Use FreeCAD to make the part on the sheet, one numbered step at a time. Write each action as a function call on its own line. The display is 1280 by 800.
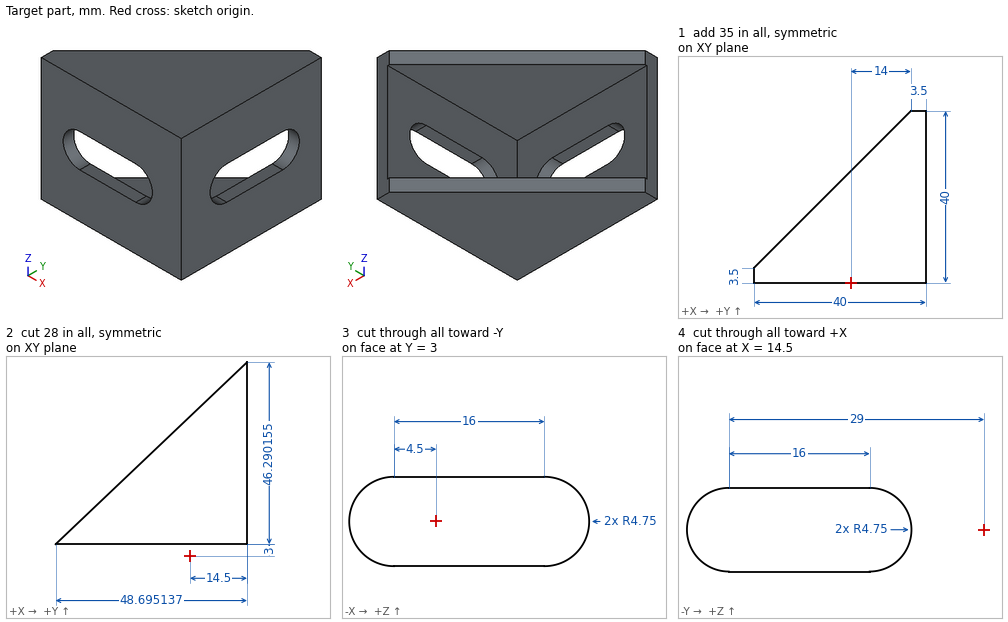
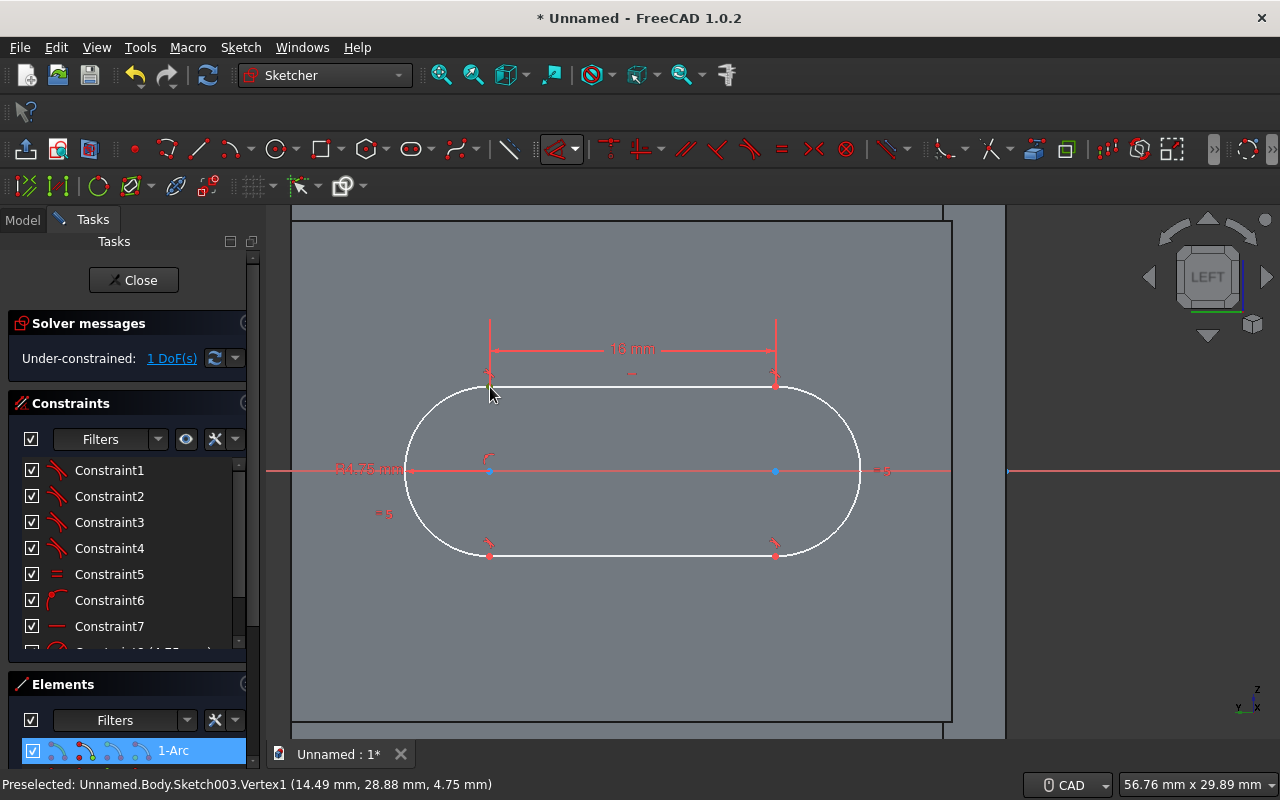
key(l)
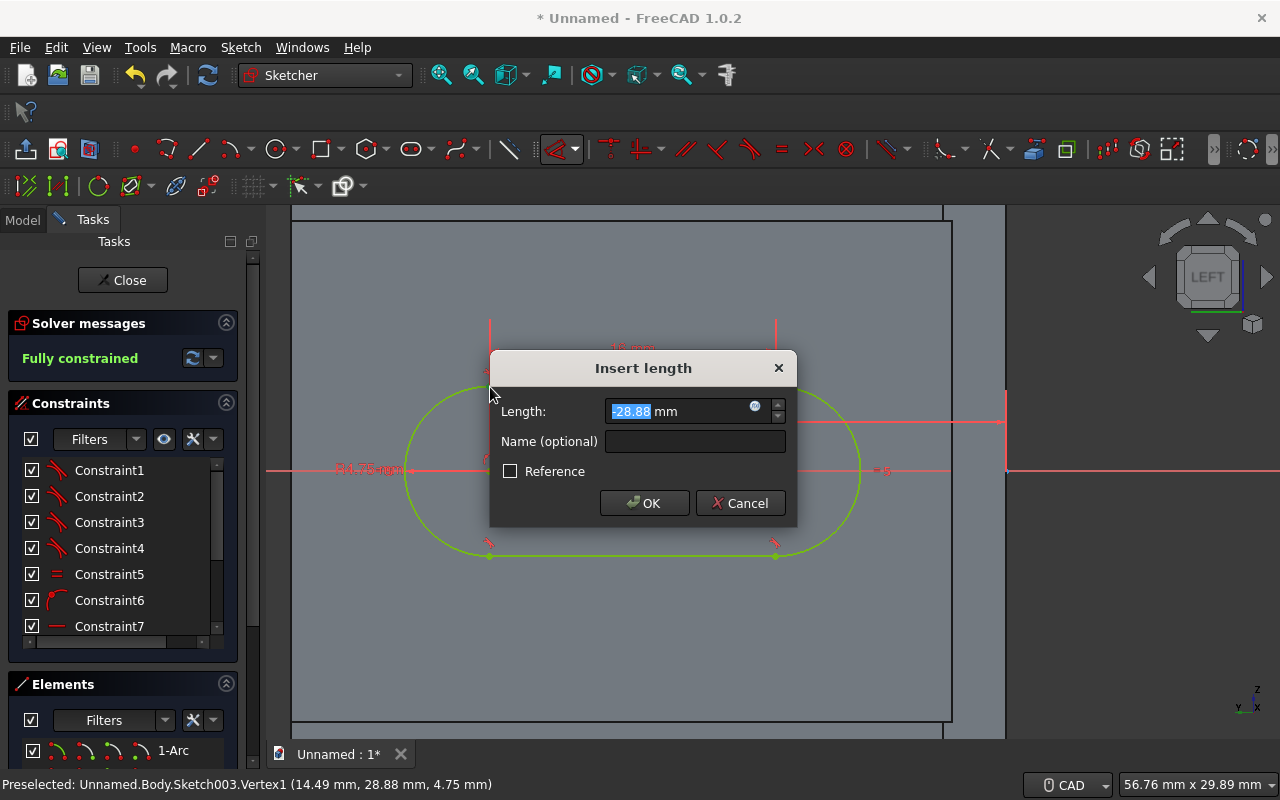
text(-29)
key(Return)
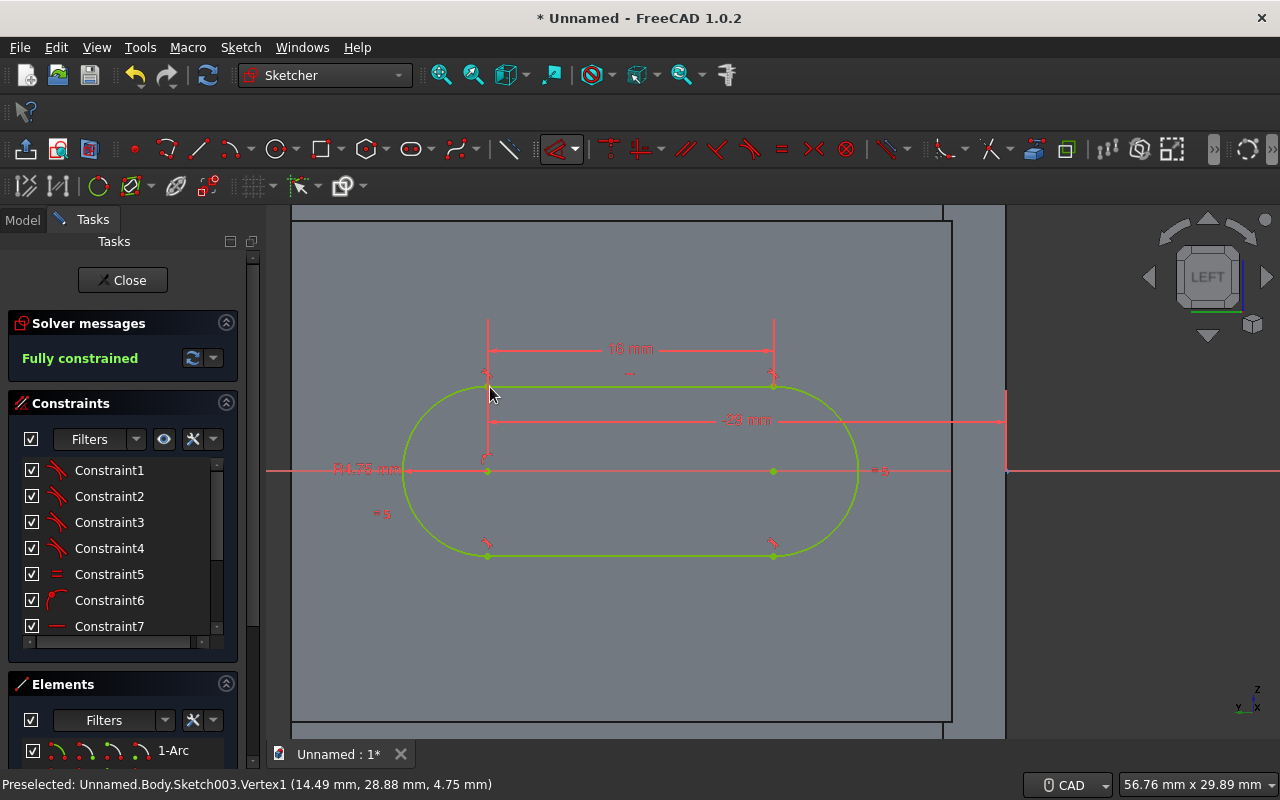
click(123, 280)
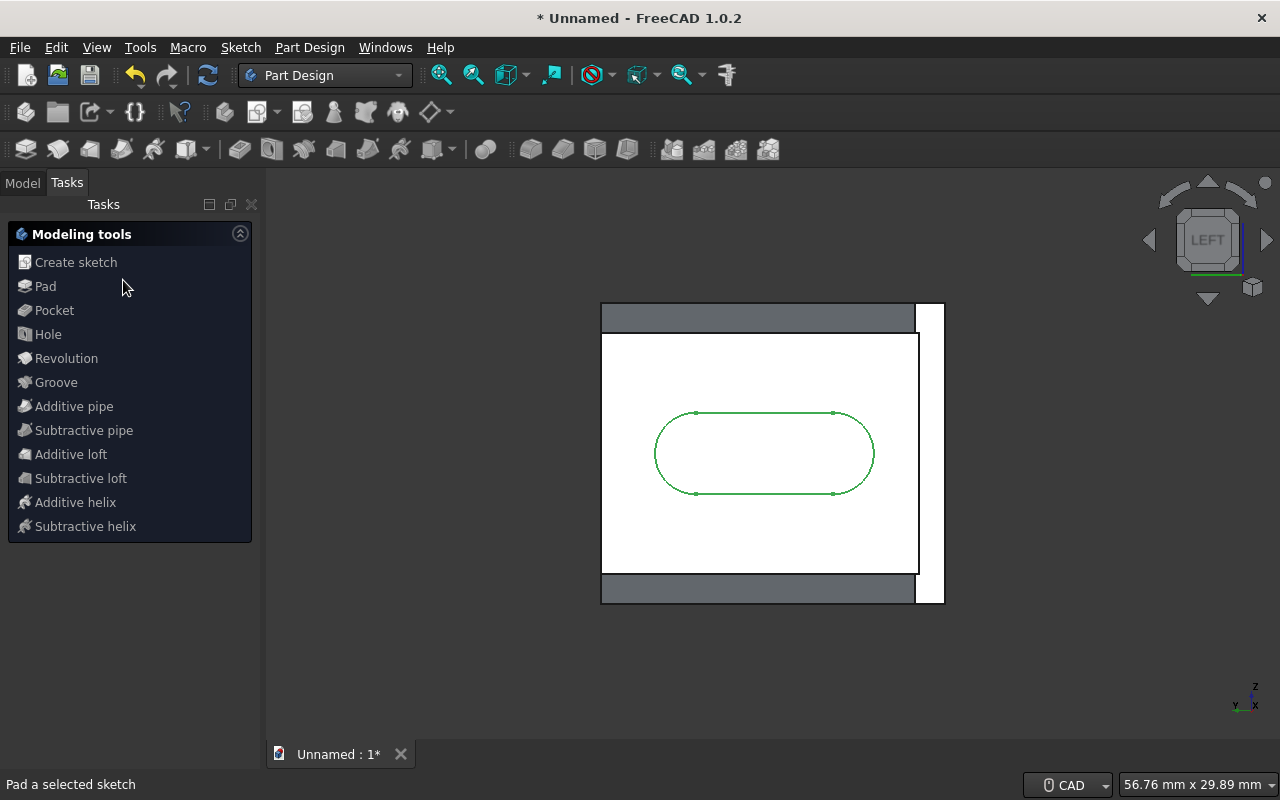
click(240, 150)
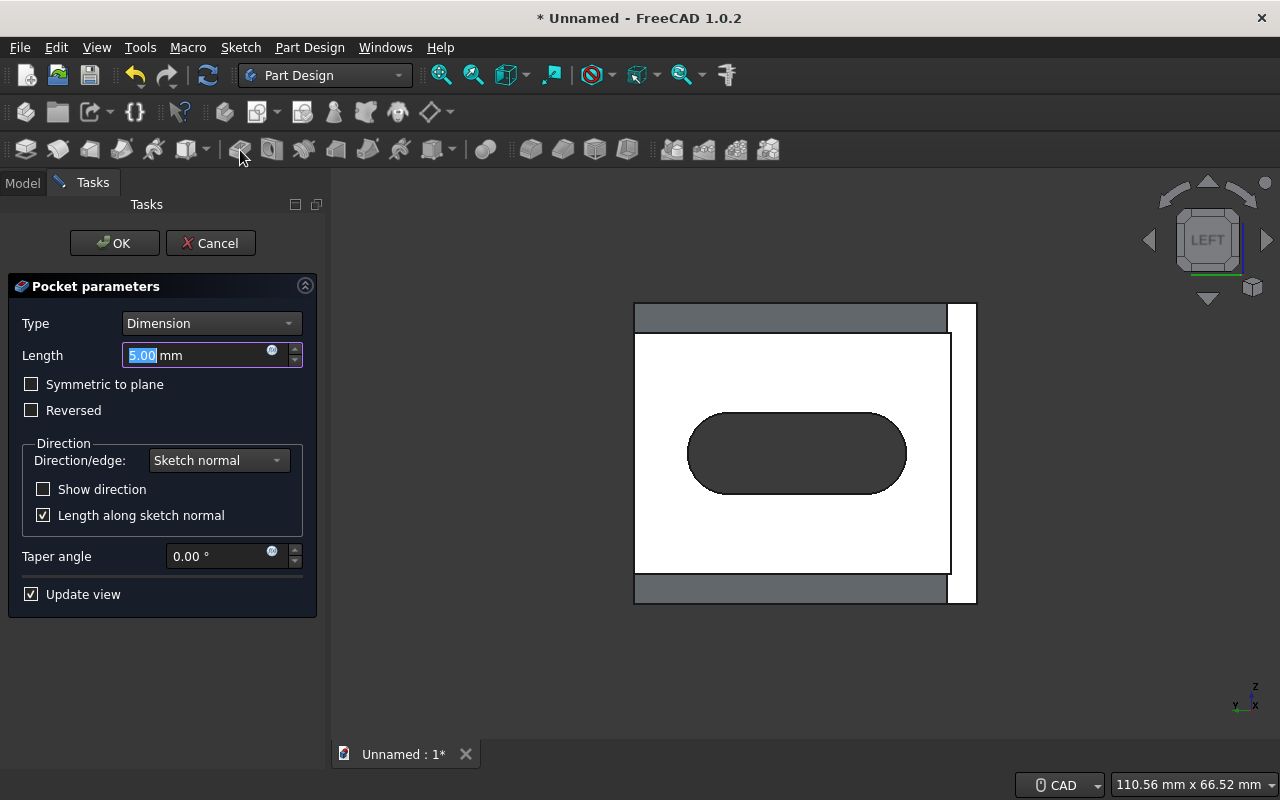
click(212, 324)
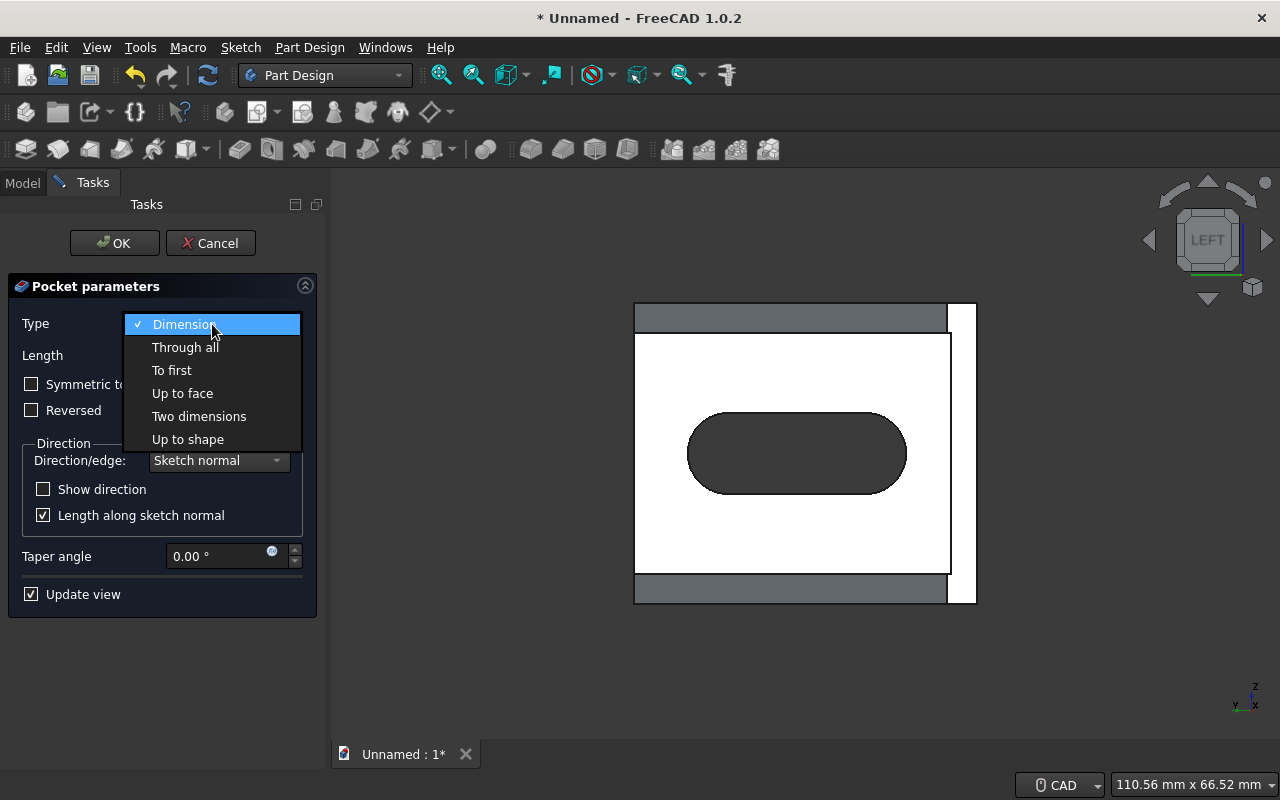
click(212, 348)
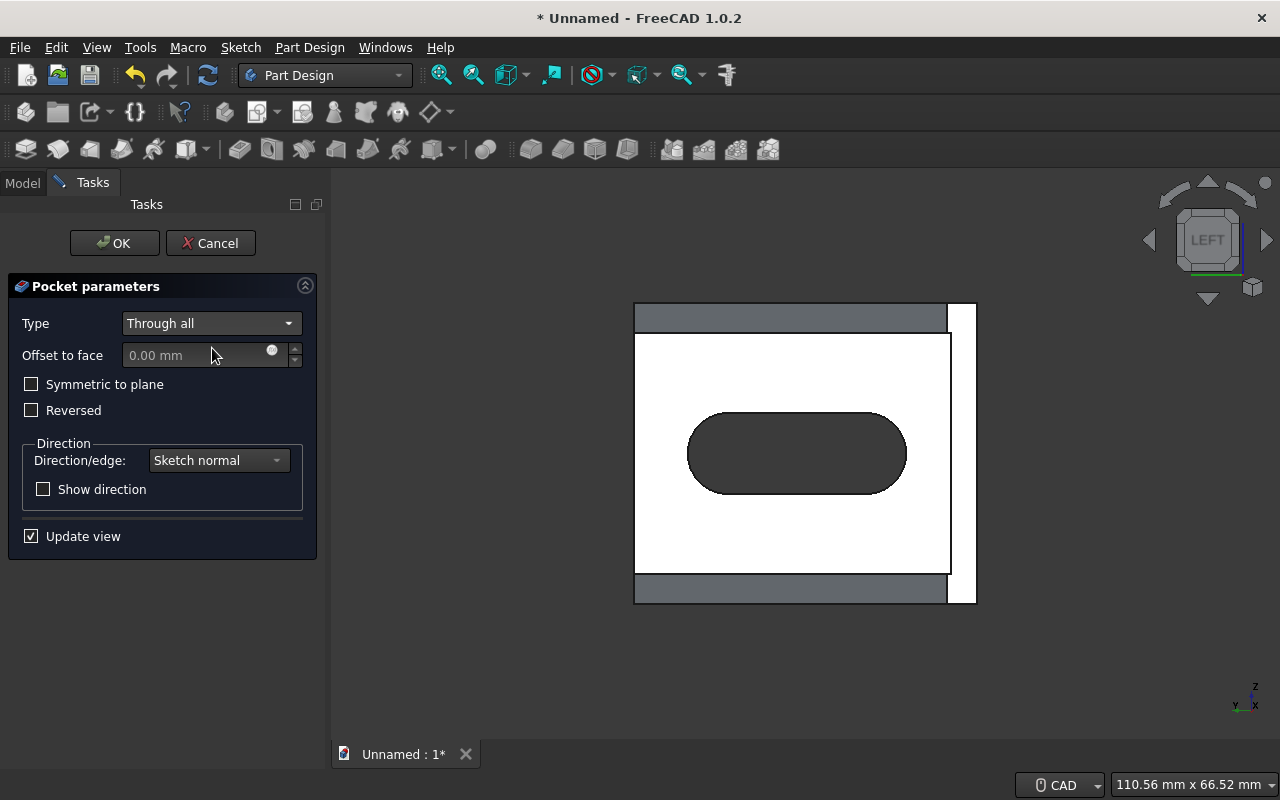
click(115, 243)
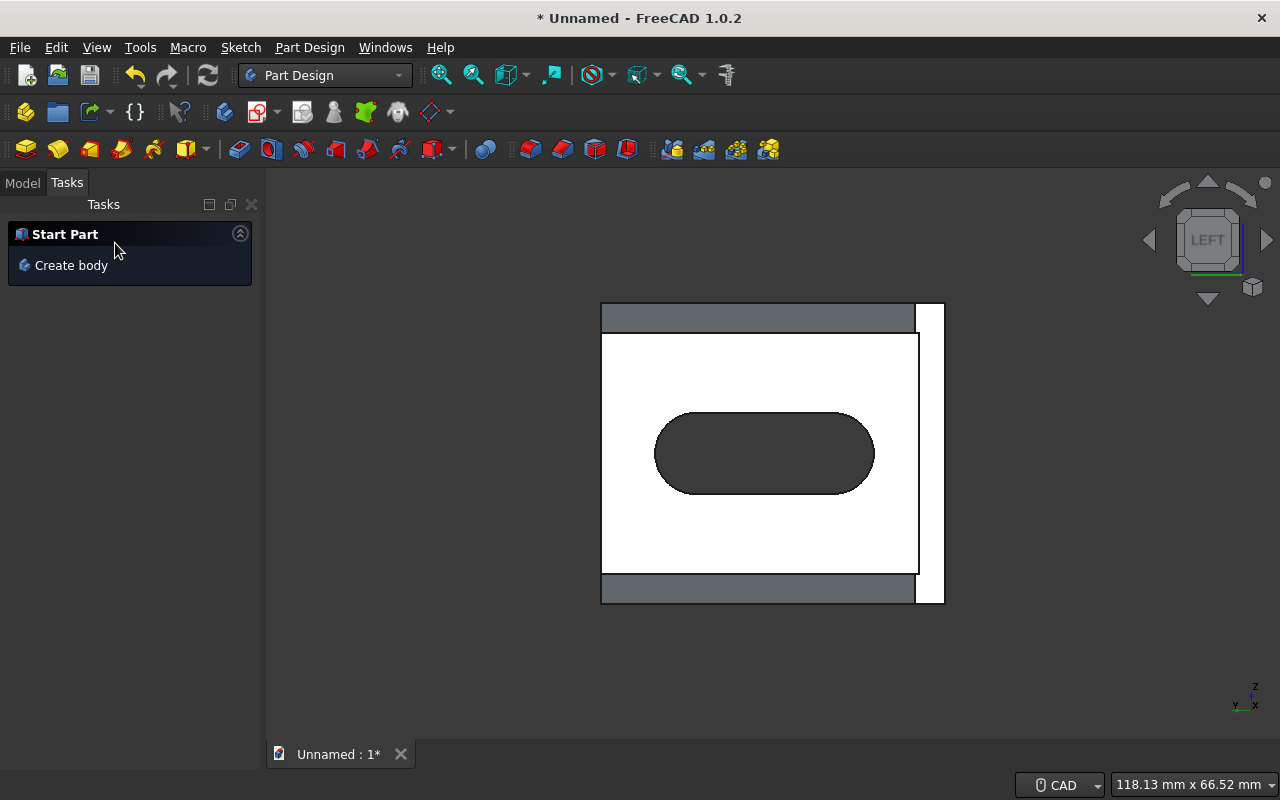
key(0)